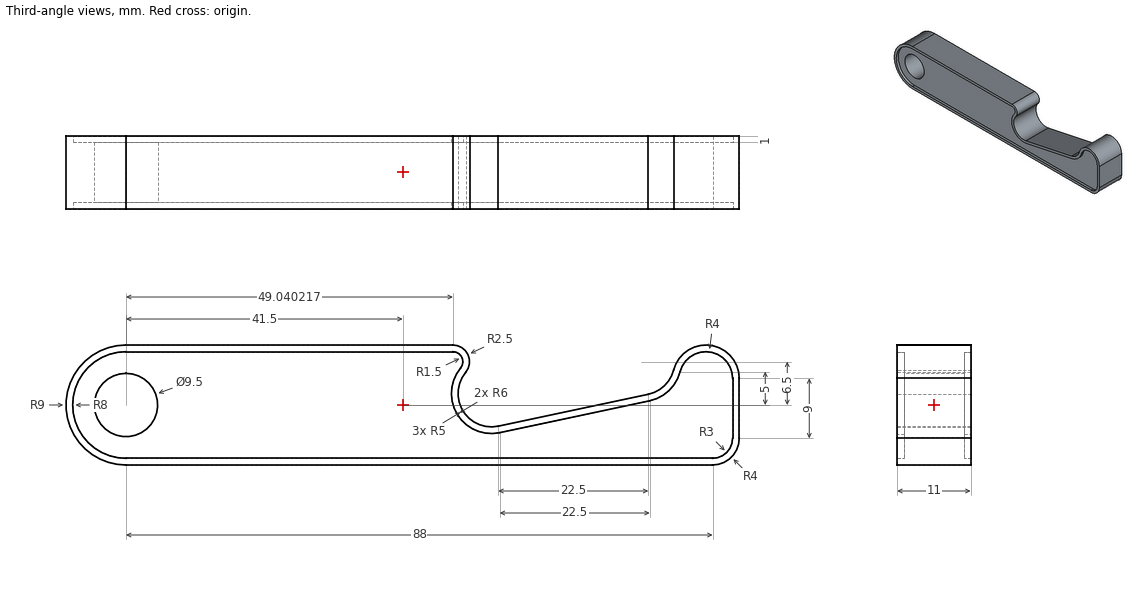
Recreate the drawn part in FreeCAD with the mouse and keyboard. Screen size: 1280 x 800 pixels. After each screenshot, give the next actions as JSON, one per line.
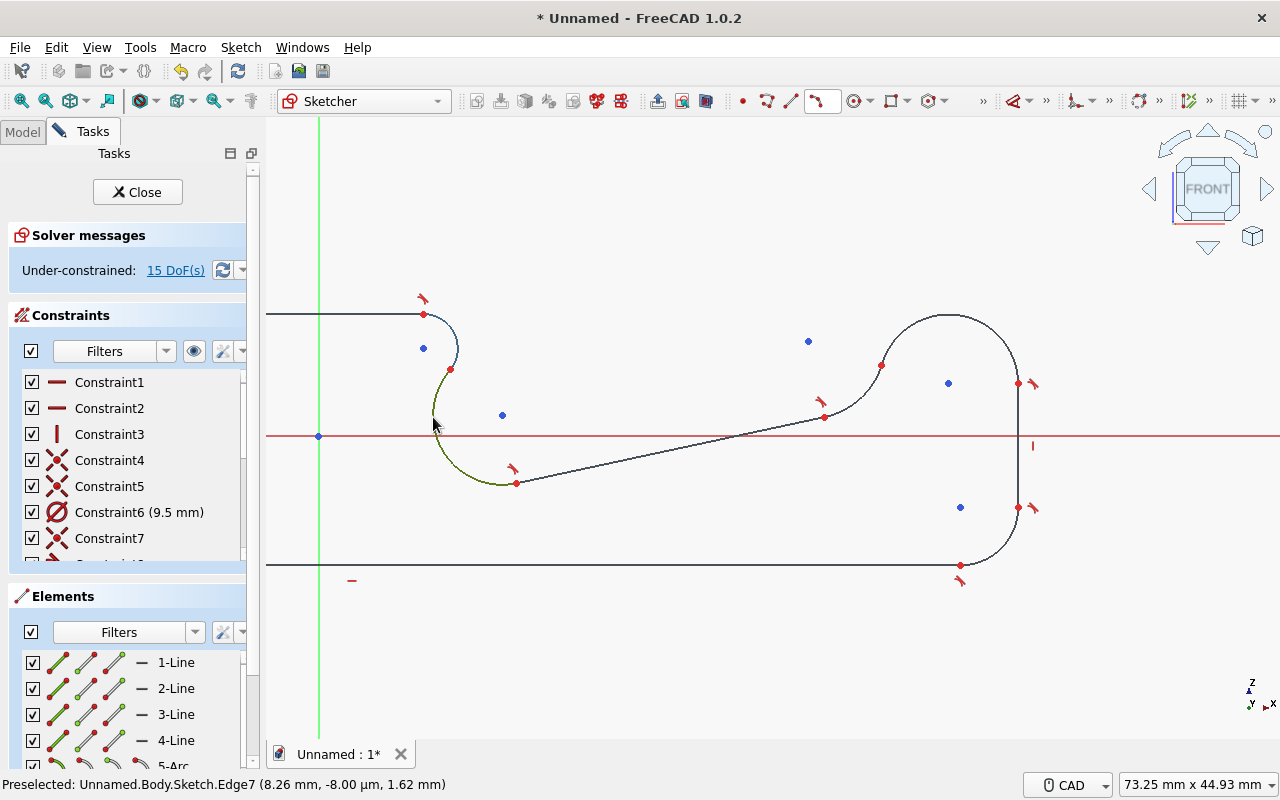
{"action": "key", "text": "t"}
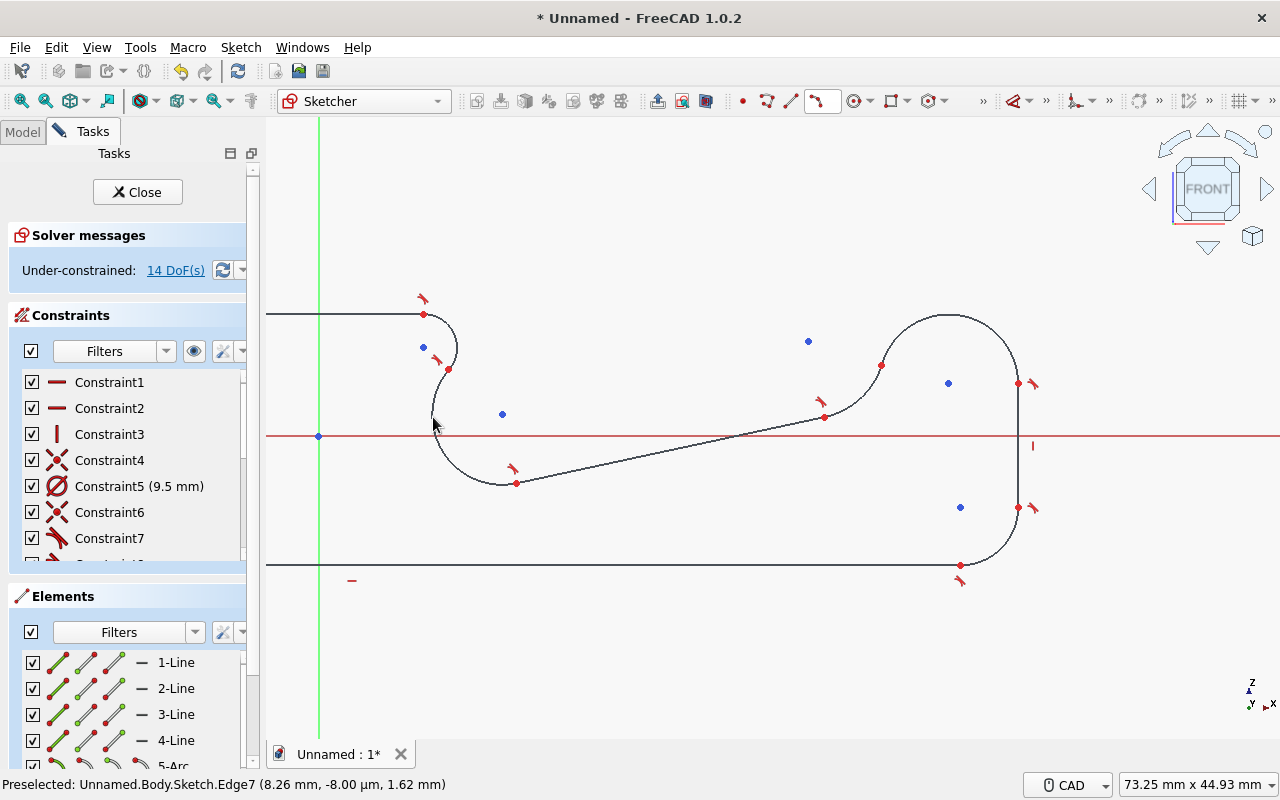
{"action": "left_click", "coordinate": [847, 408]}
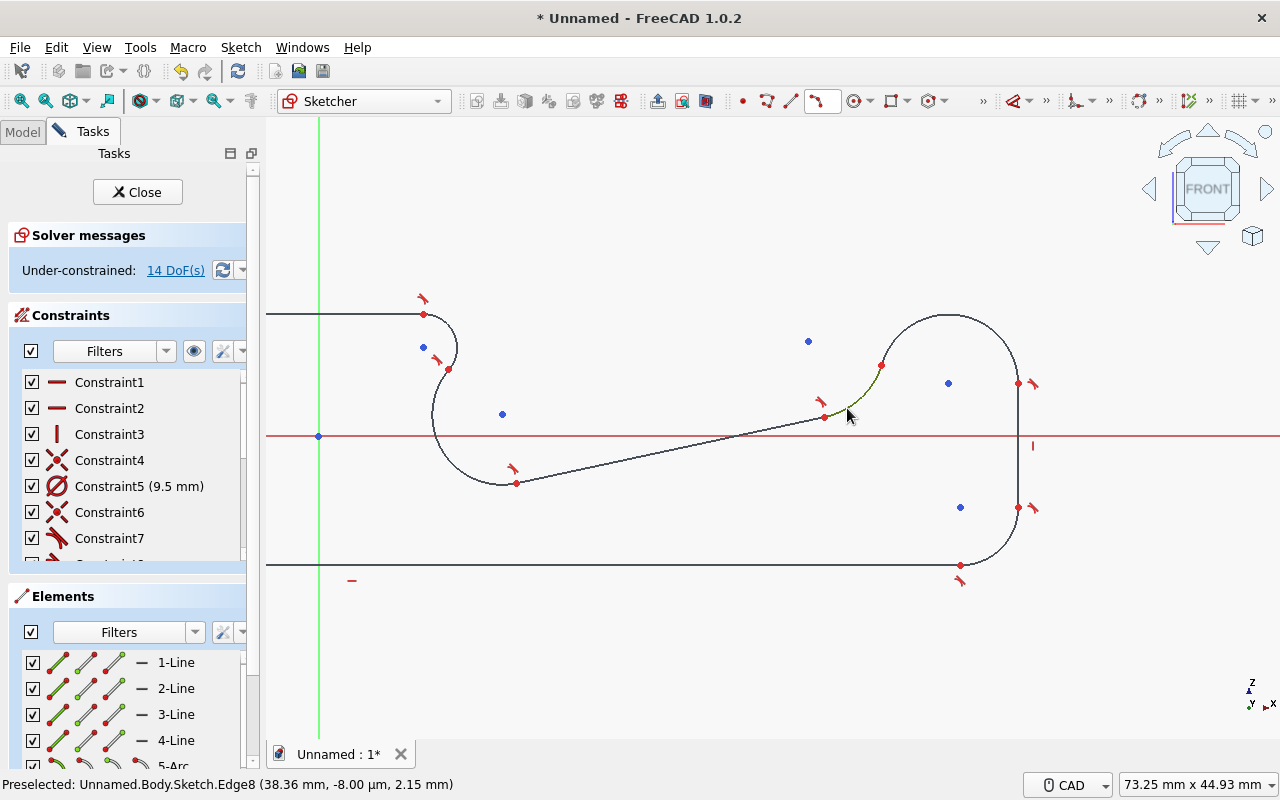
{"action": "left_click", "coordinate": [994, 331]}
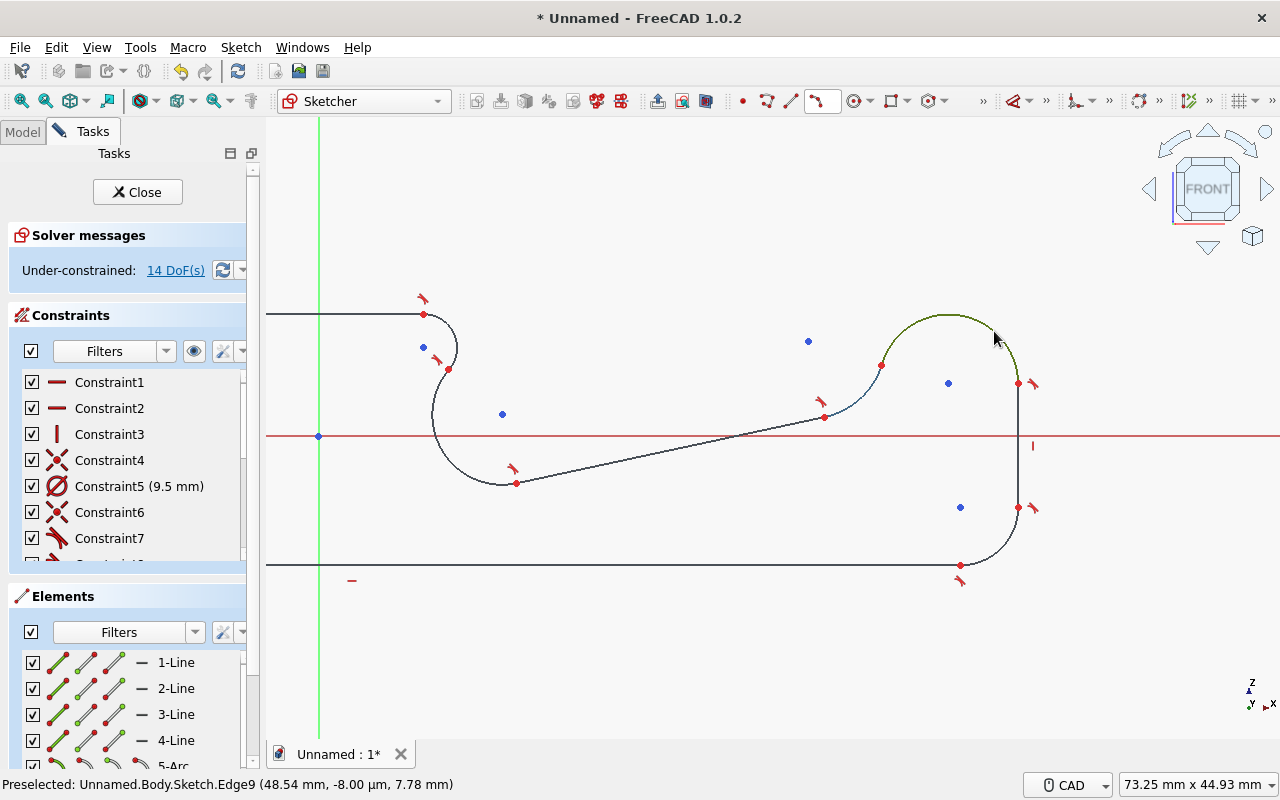
{"action": "key", "text": "t"}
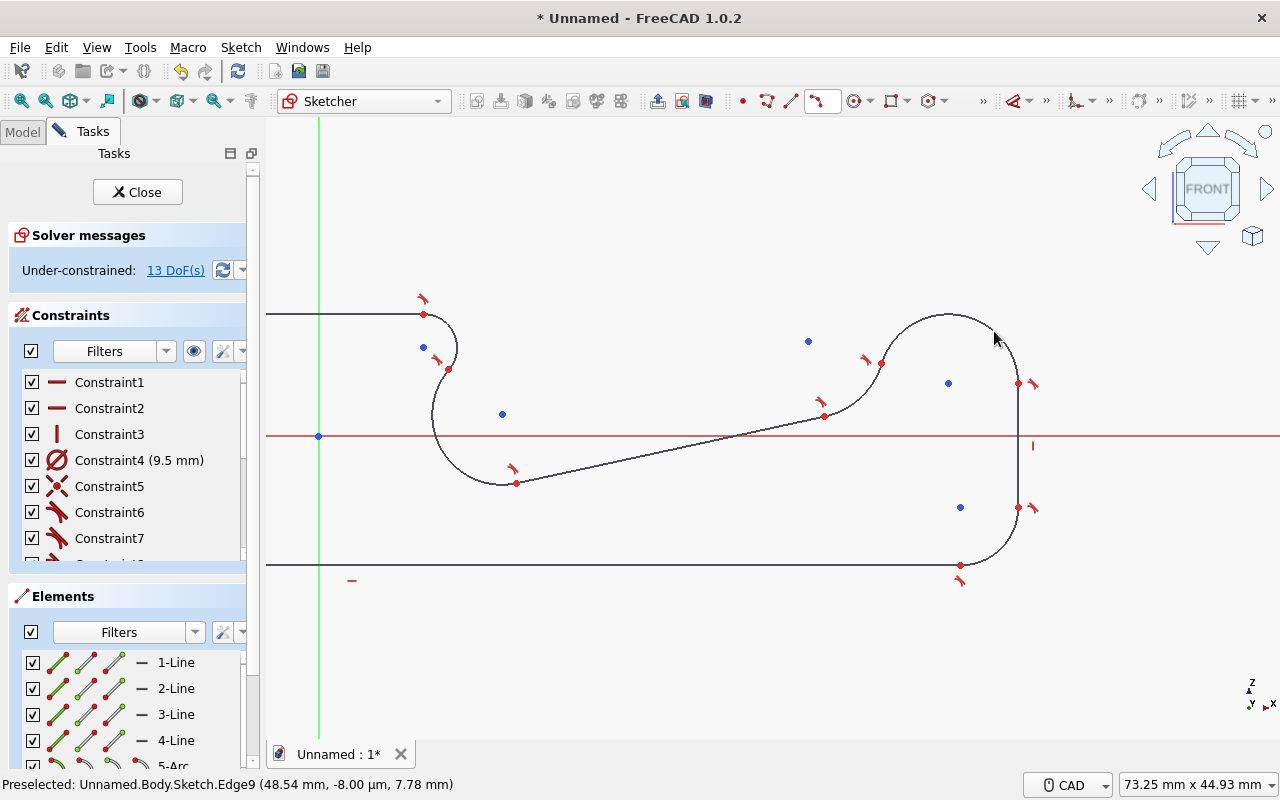
{"action": "left_click", "coordinate": [432, 418]}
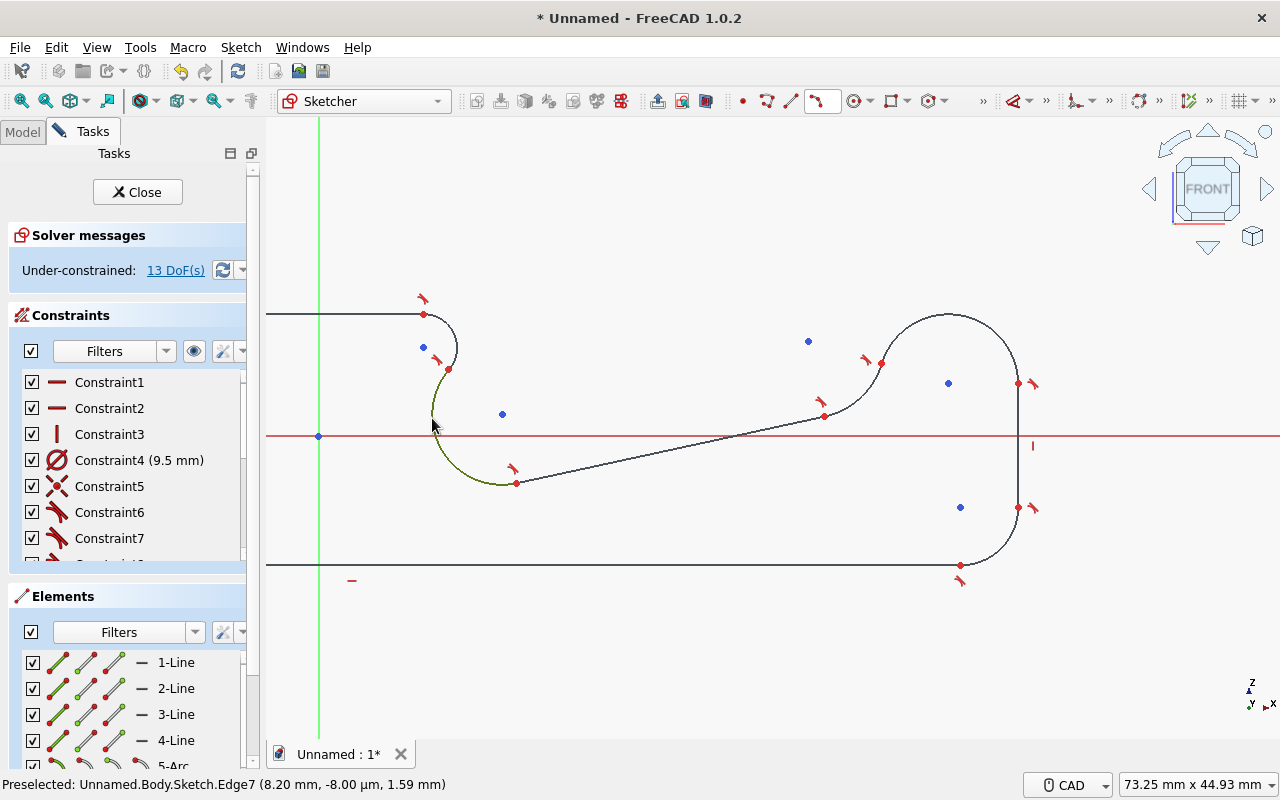
{"action": "left_click", "coordinate": [847, 408]}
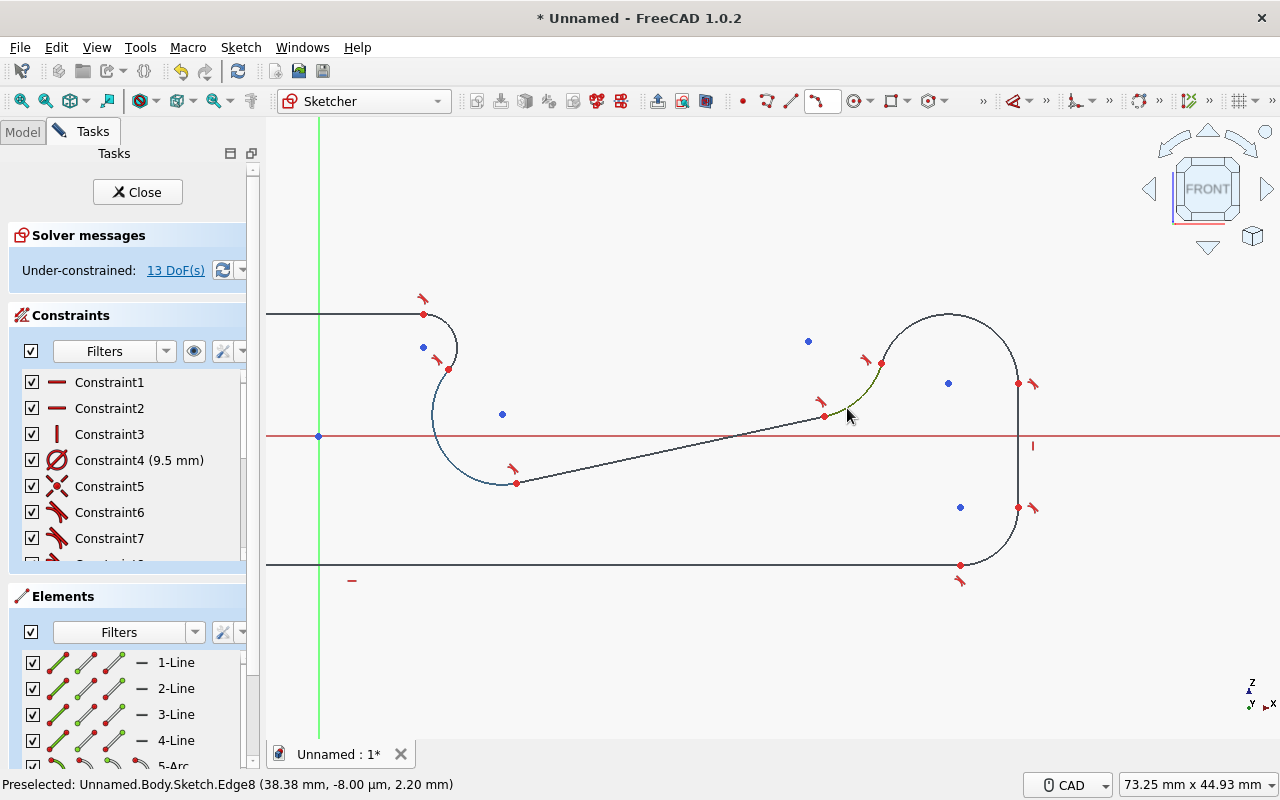
{"action": "left_click", "coordinate": [994, 331]}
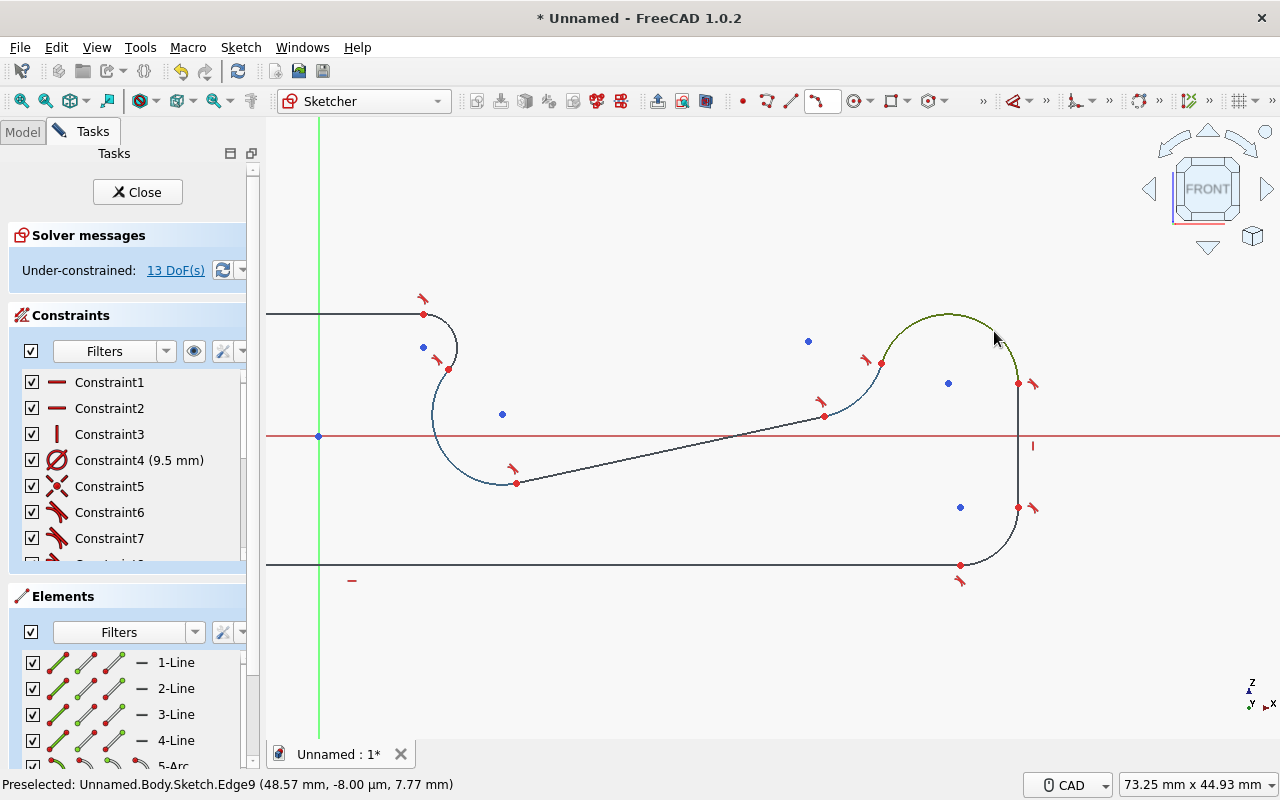
{"action": "key", "text": "e"}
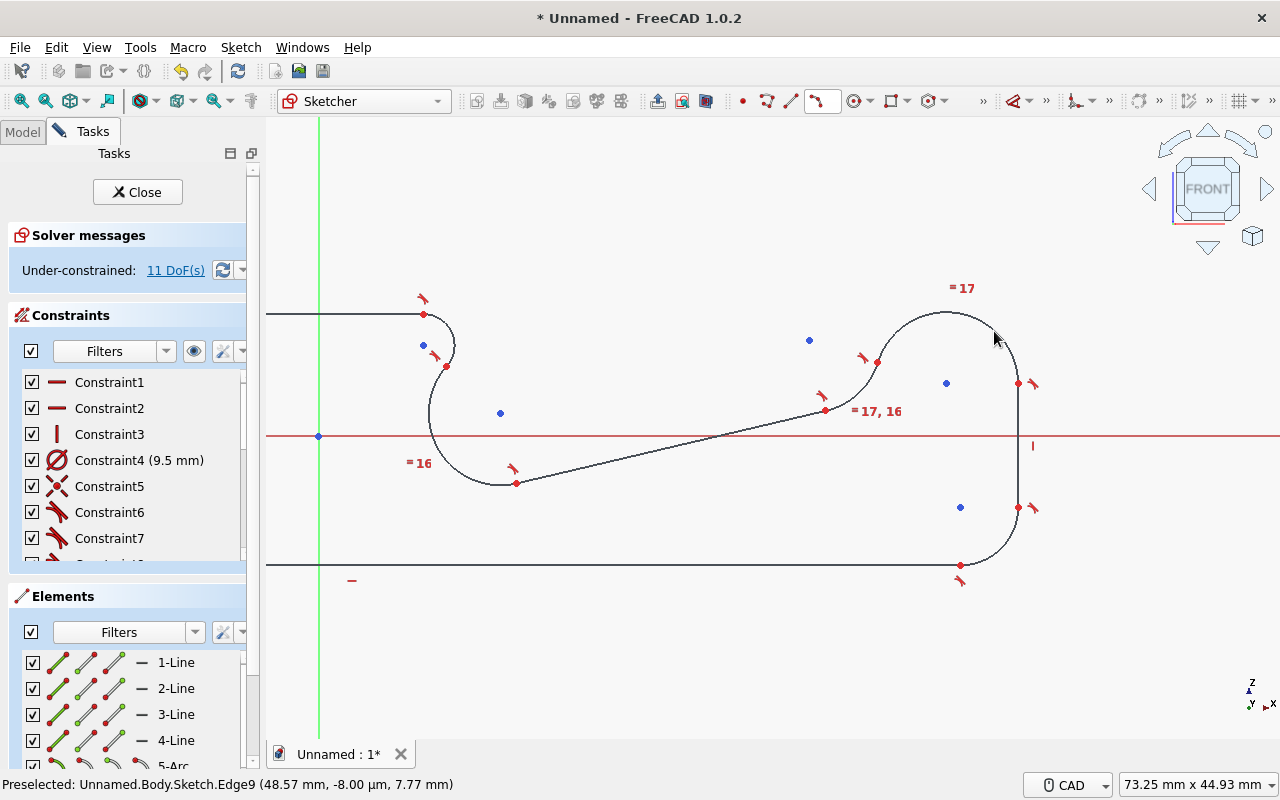
{"action": "scroll", "coordinate": [1019, 421], "scroll_direction": "down", "scroll_amount": 4}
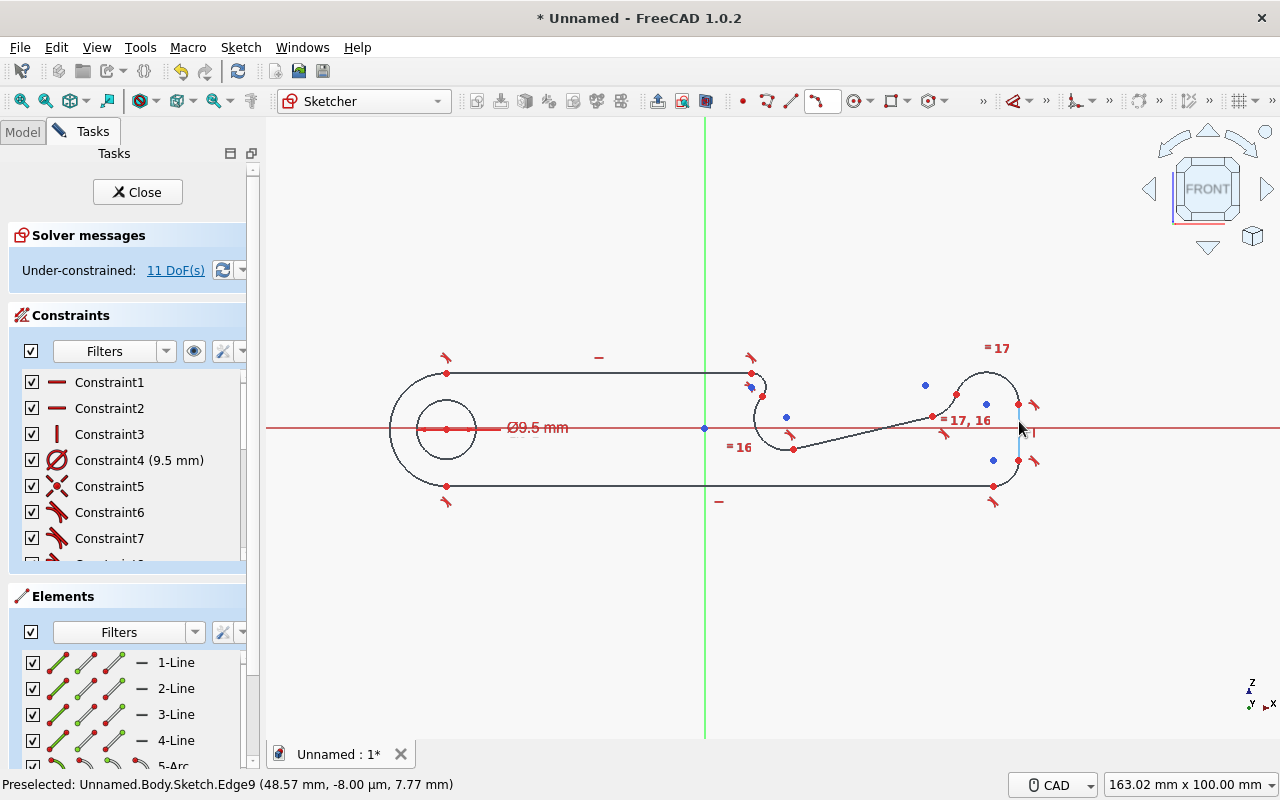
{"action": "left_click", "coordinate": [446, 430]}